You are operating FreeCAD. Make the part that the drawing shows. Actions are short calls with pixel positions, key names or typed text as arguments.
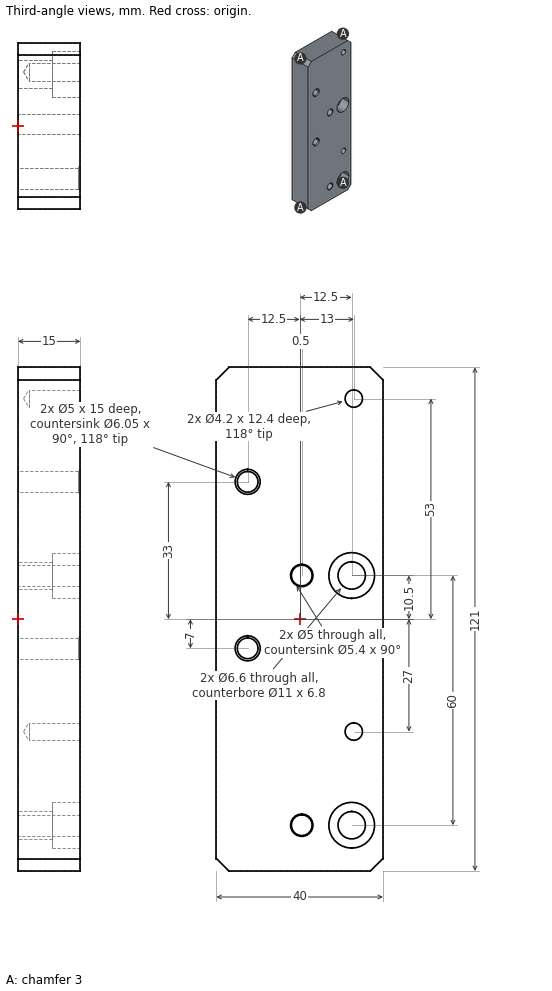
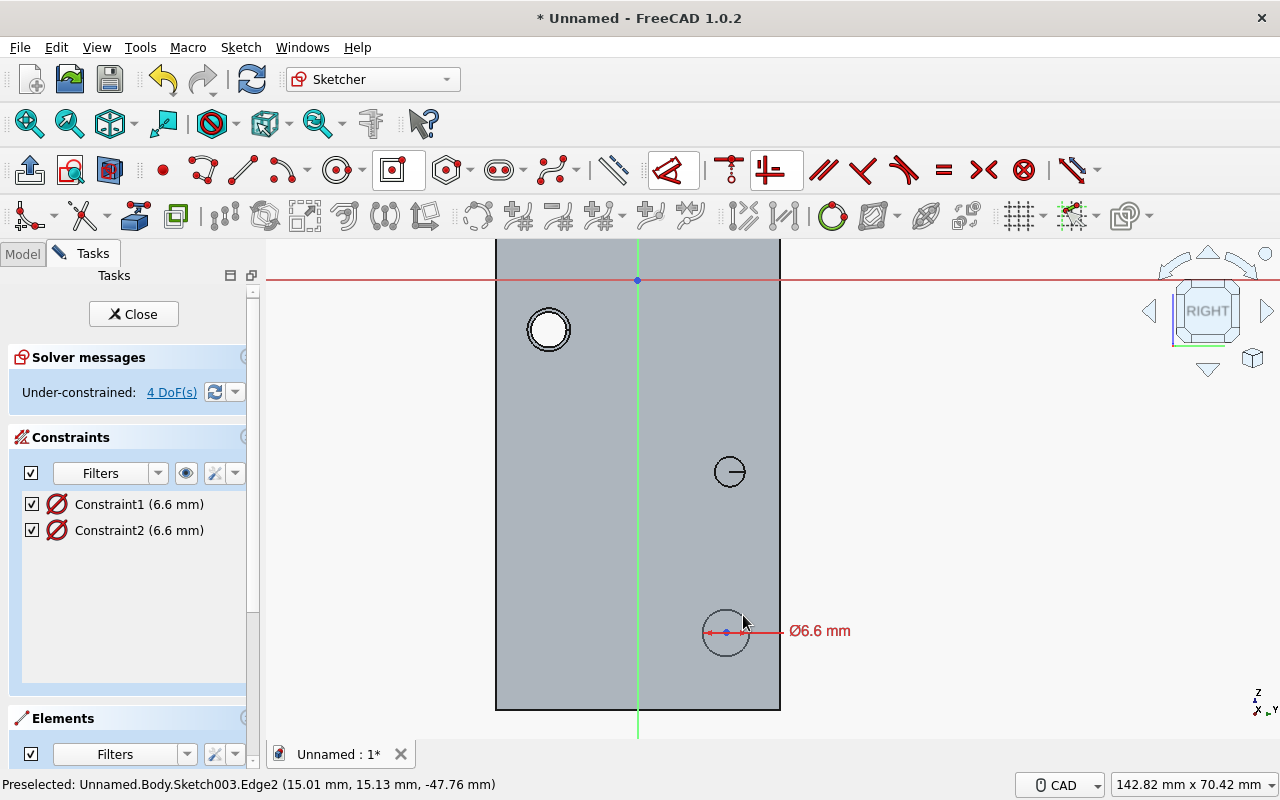
scroll(727, 632, down, 2)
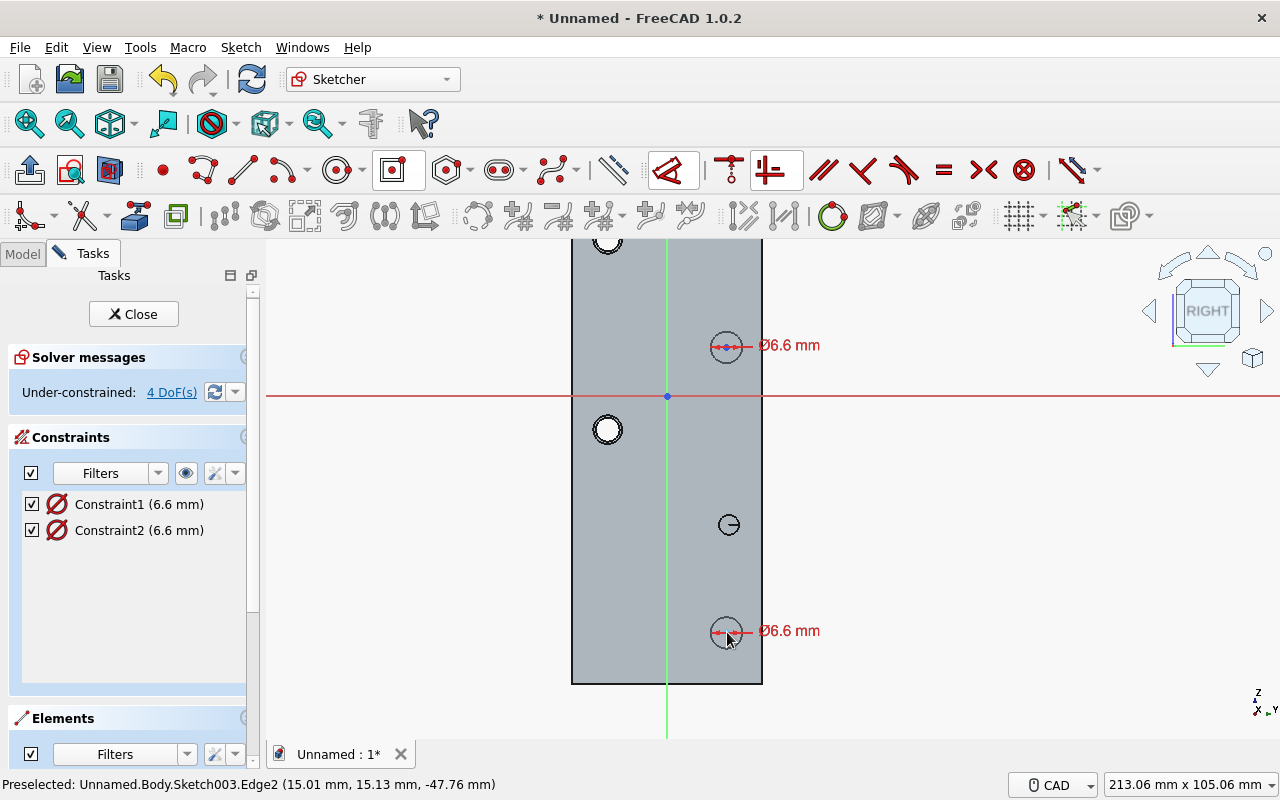
click(726, 347)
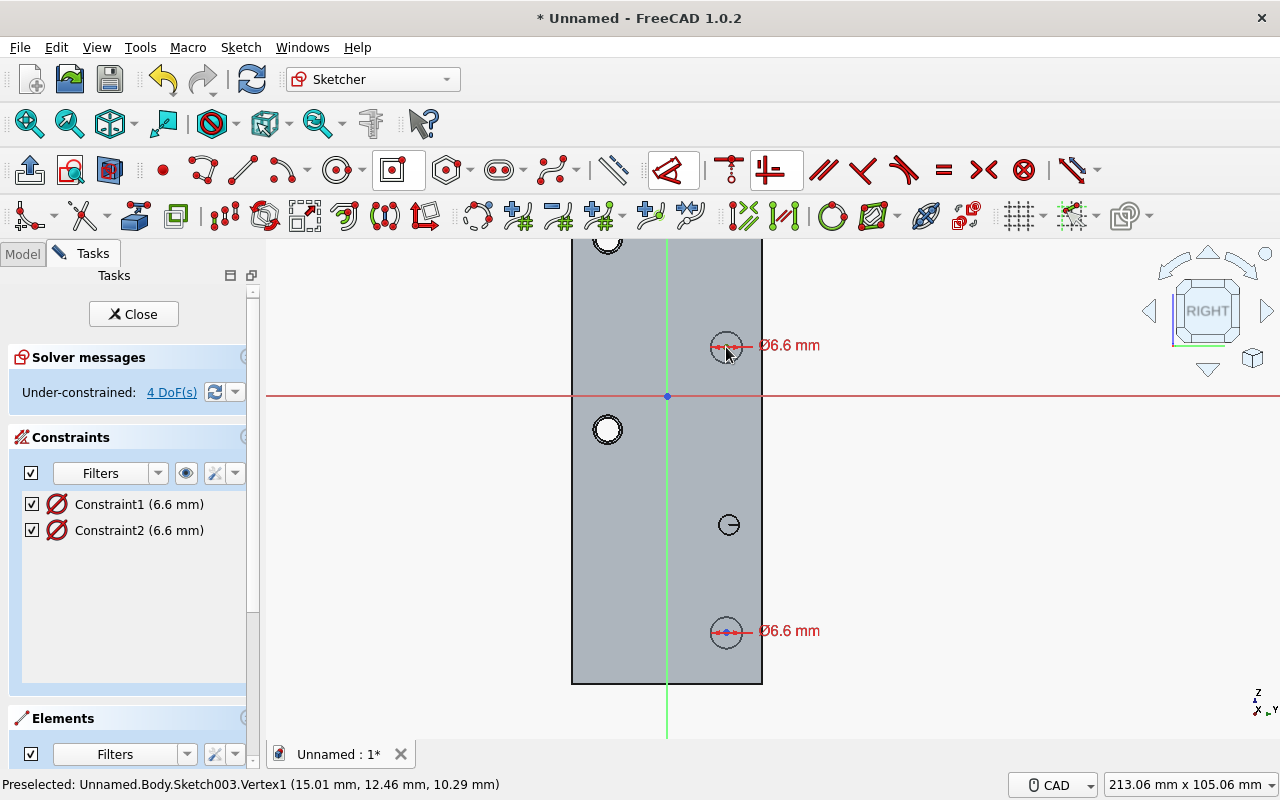
click(726, 633)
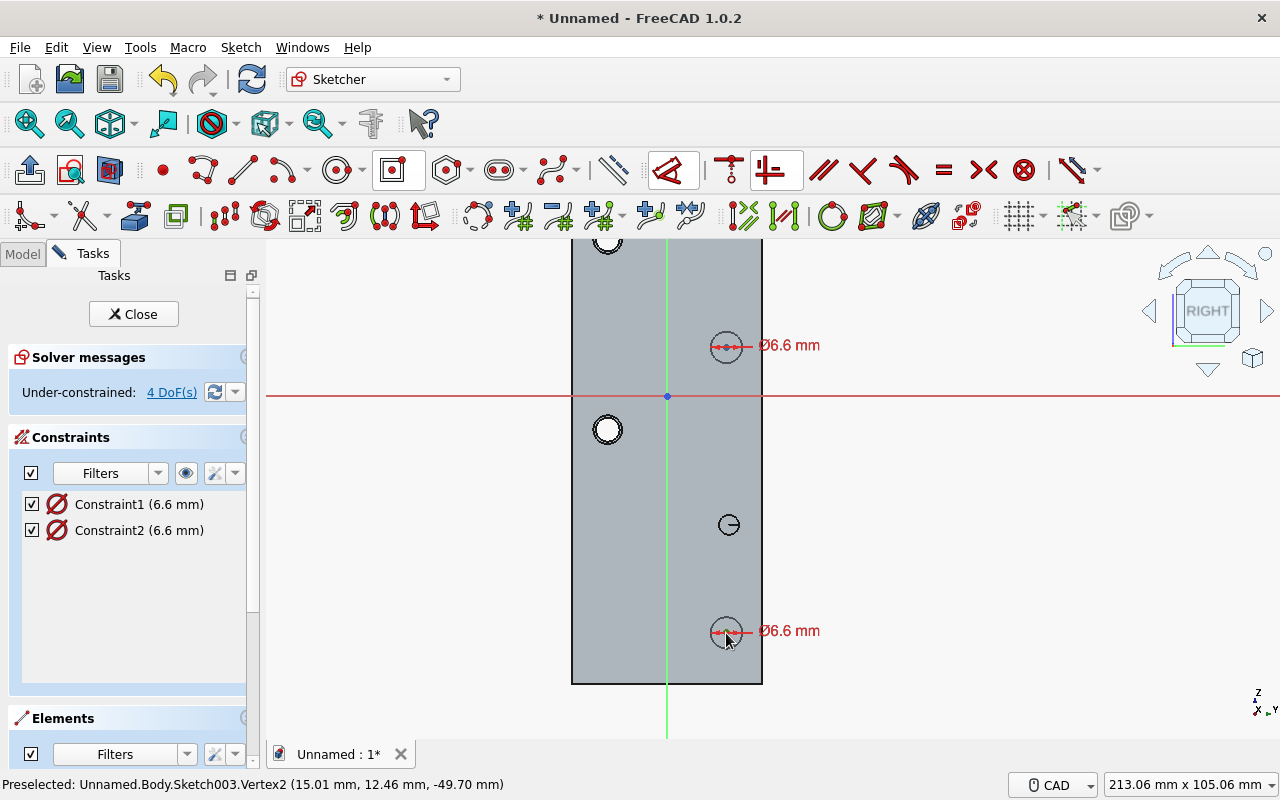
key(v)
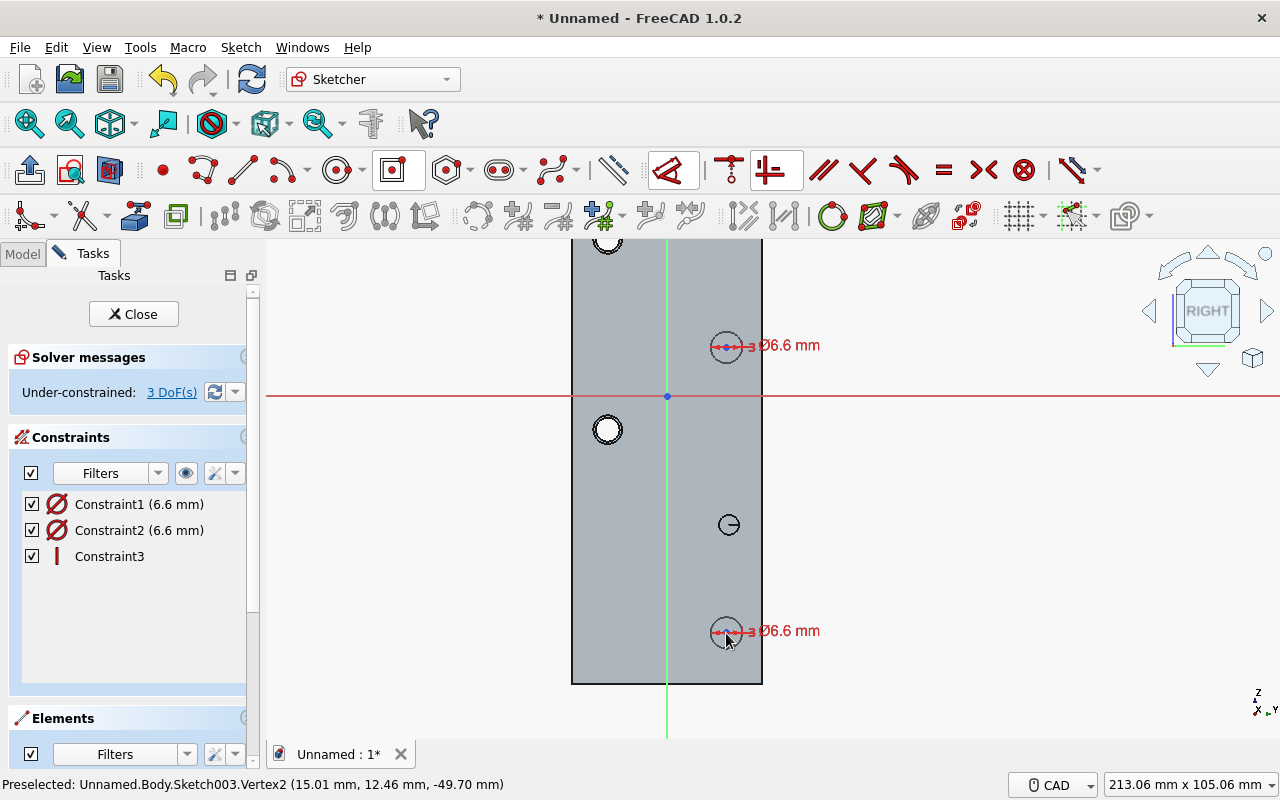
click(726, 347)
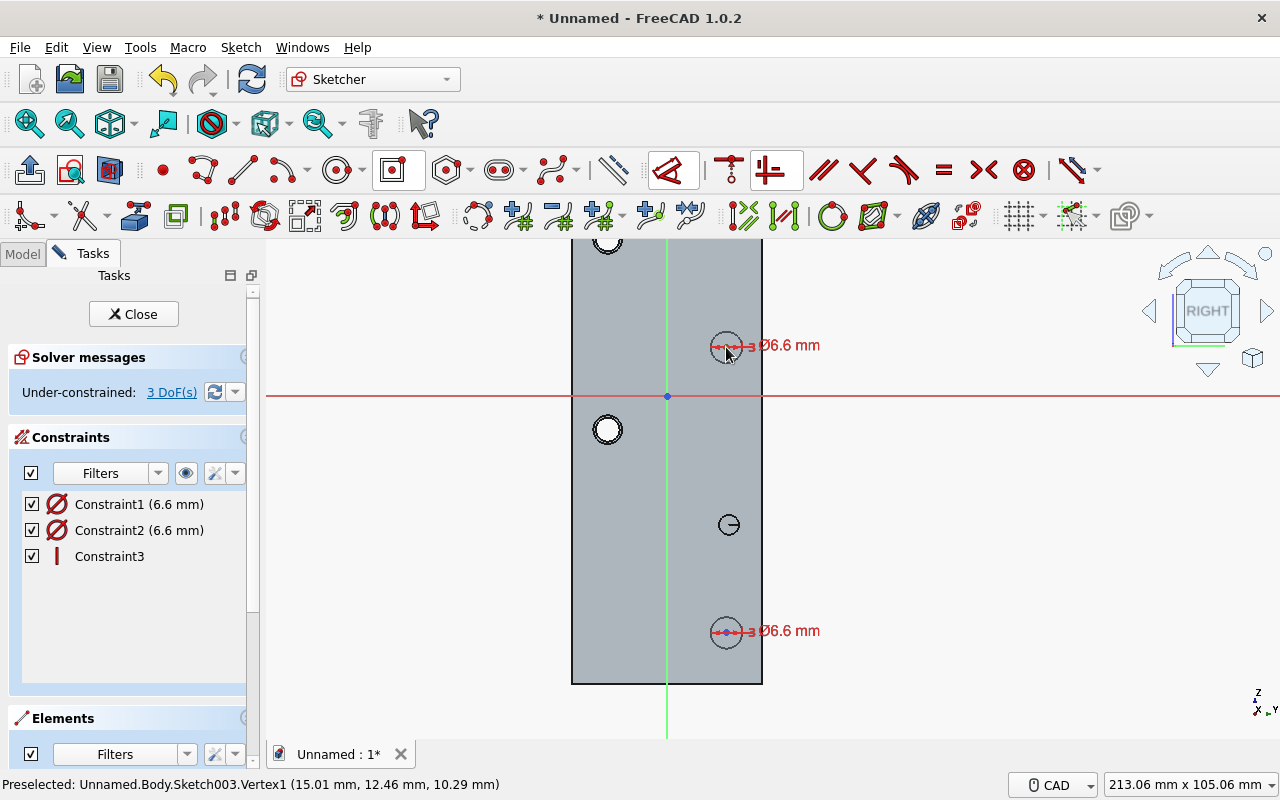
click(726, 633)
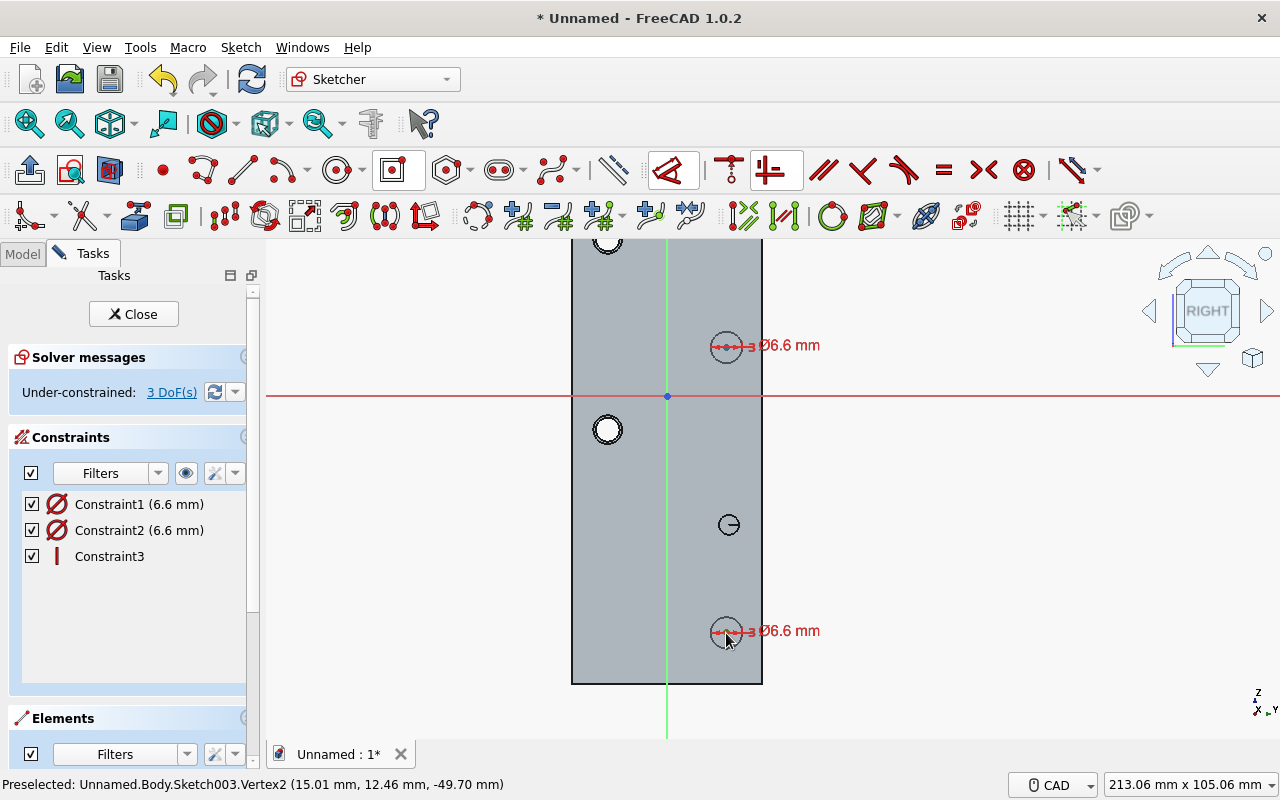
click(694, 170)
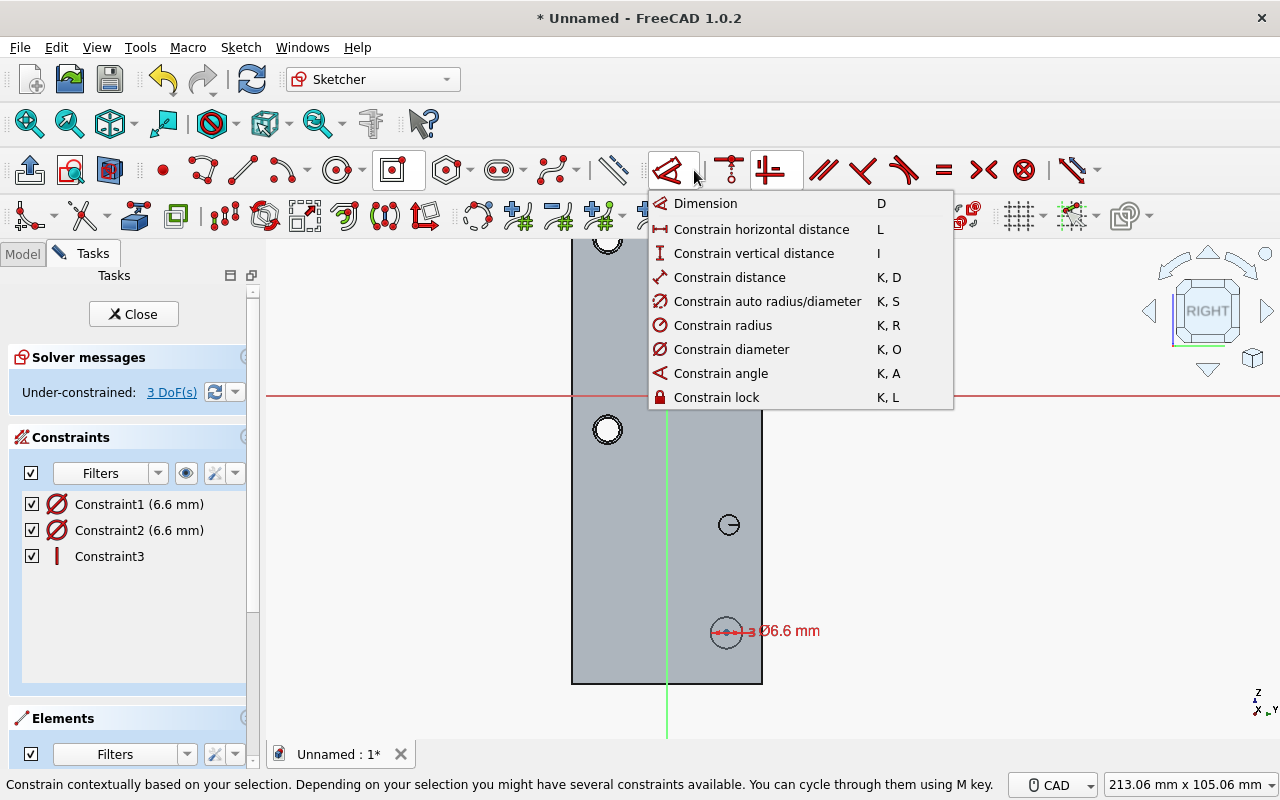
click(801, 253)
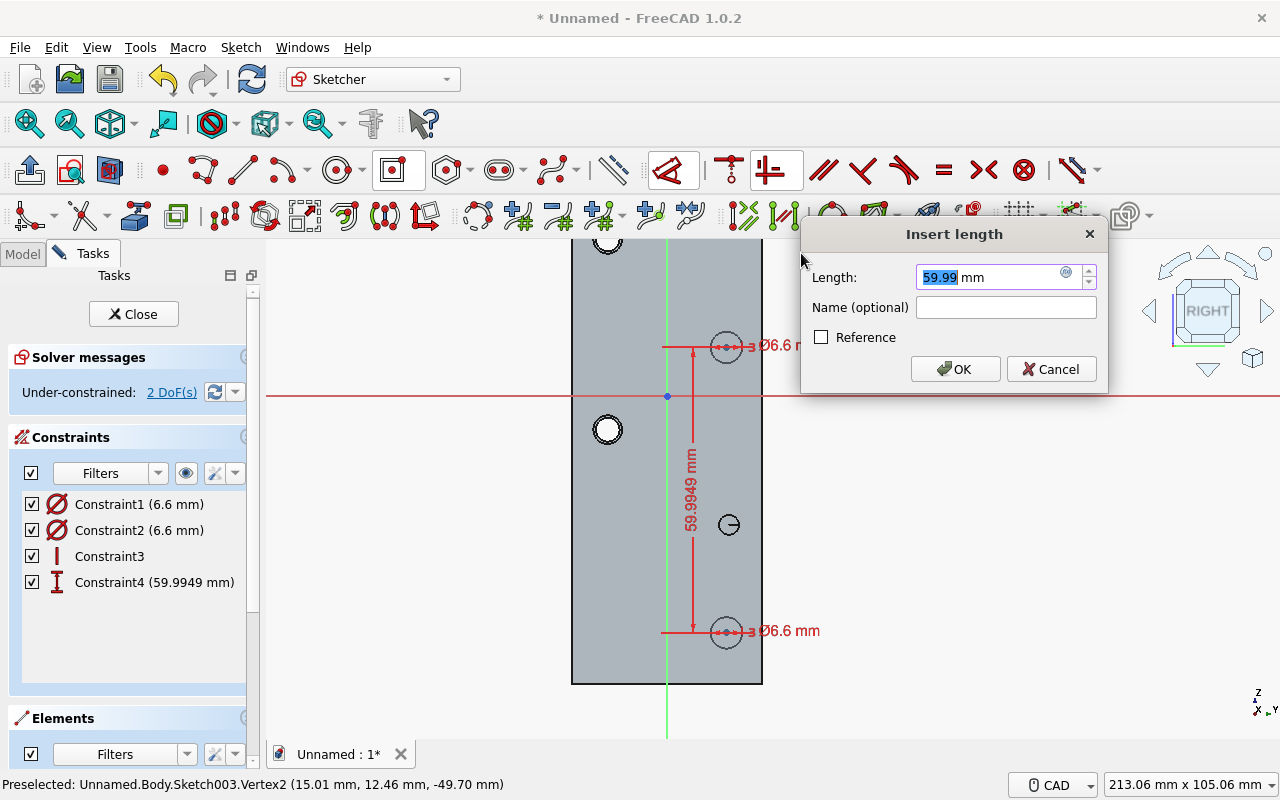
text(60)
key(Return)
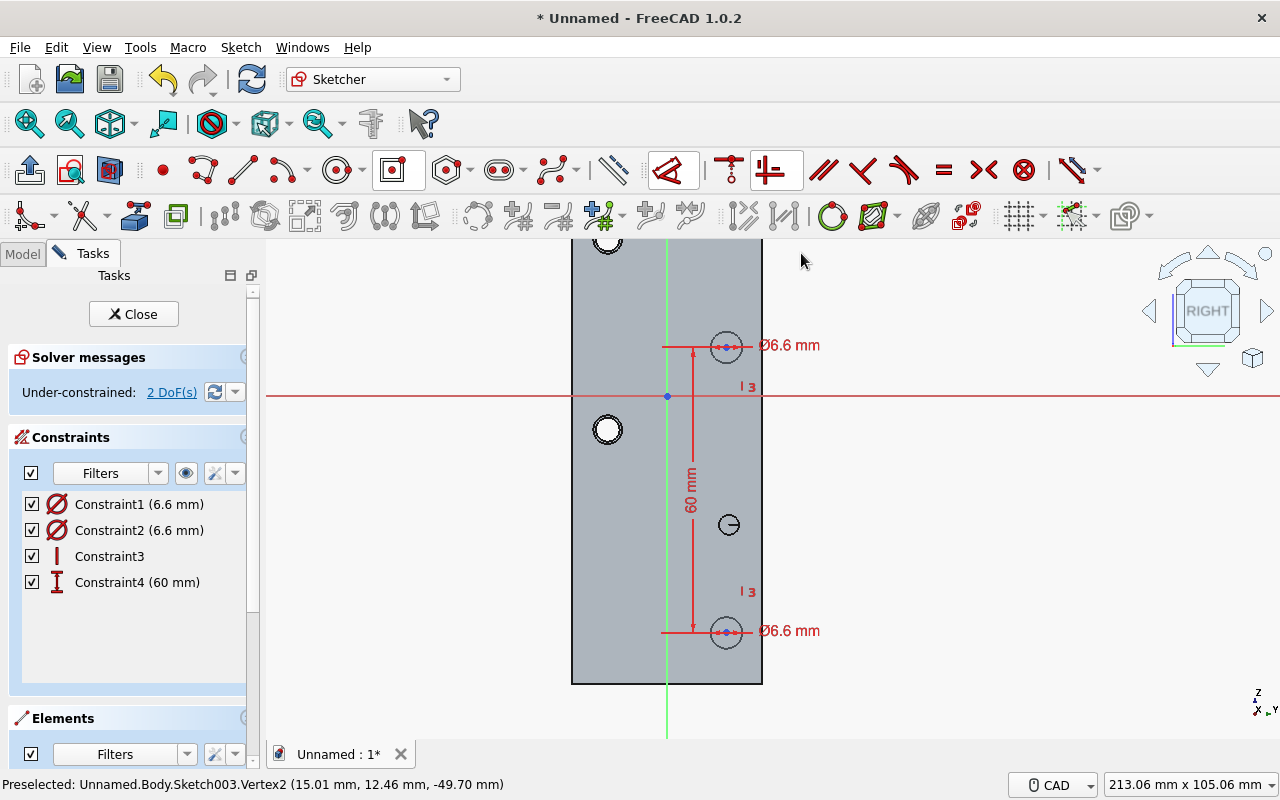
click(726, 347)